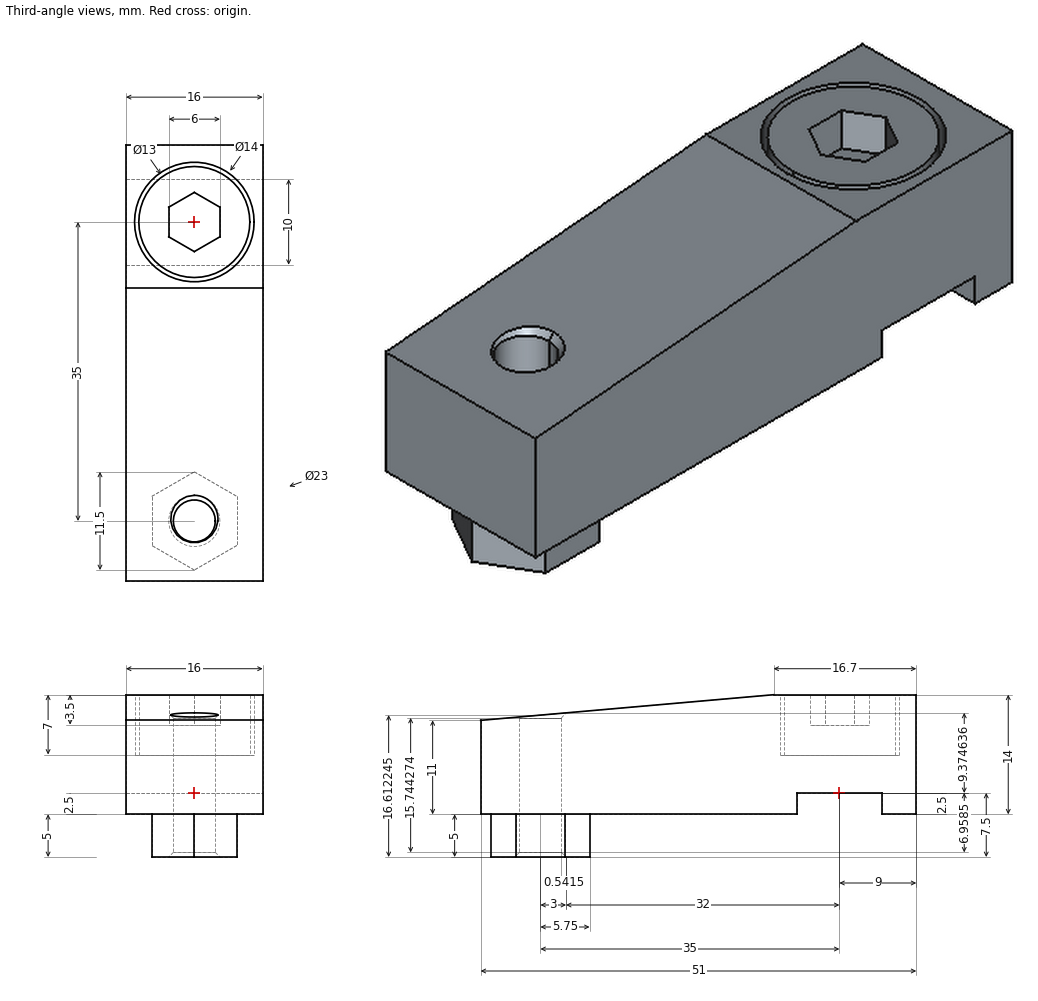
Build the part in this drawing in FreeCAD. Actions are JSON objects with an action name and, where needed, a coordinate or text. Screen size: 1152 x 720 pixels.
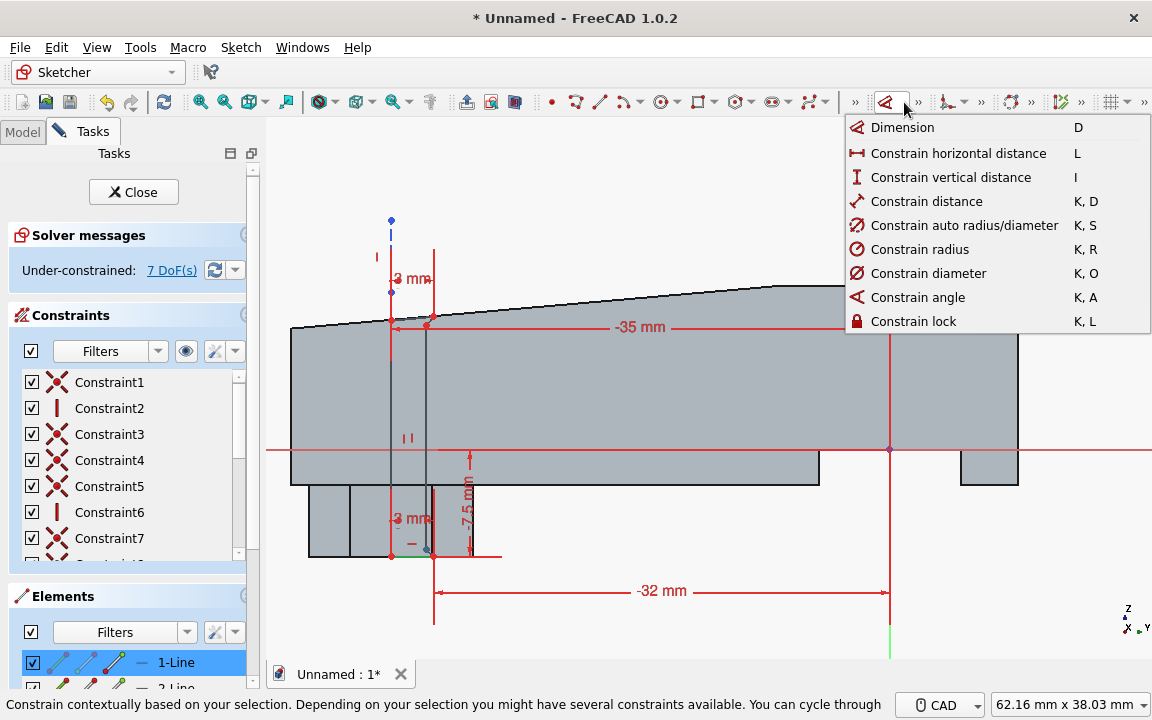
{"action": "left_click", "coordinate": [998, 177]}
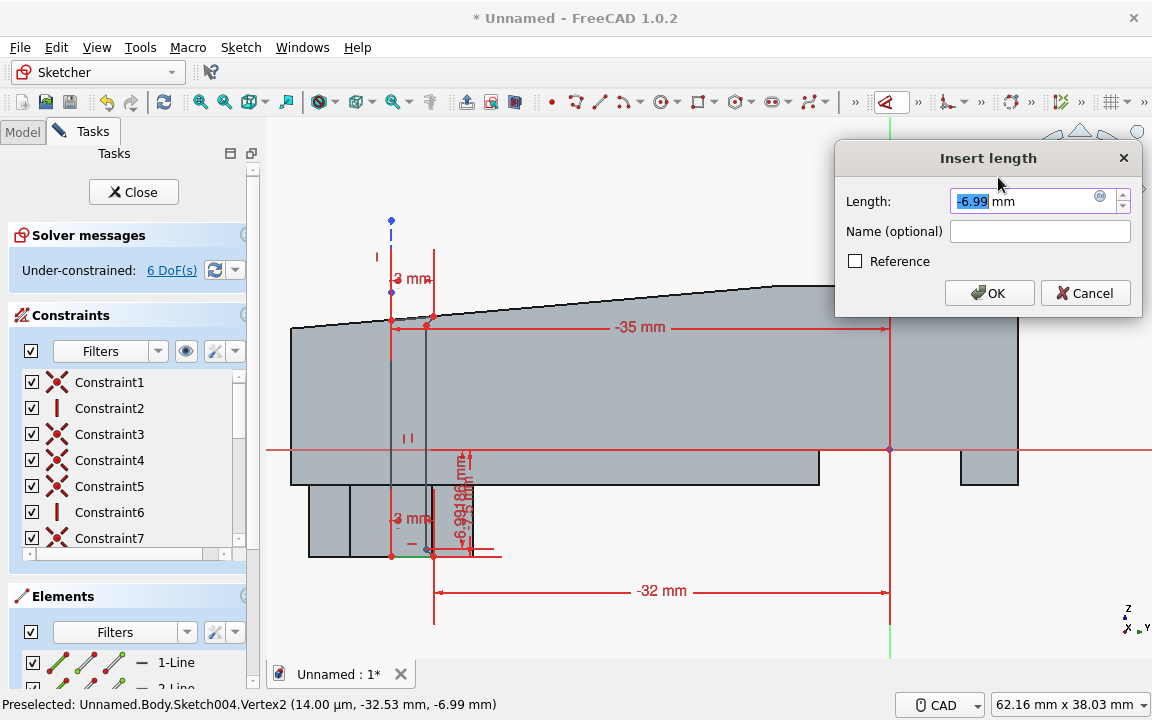
{"action": "type", "text": "-6.9585"}
{"action": "key", "text": "Return"}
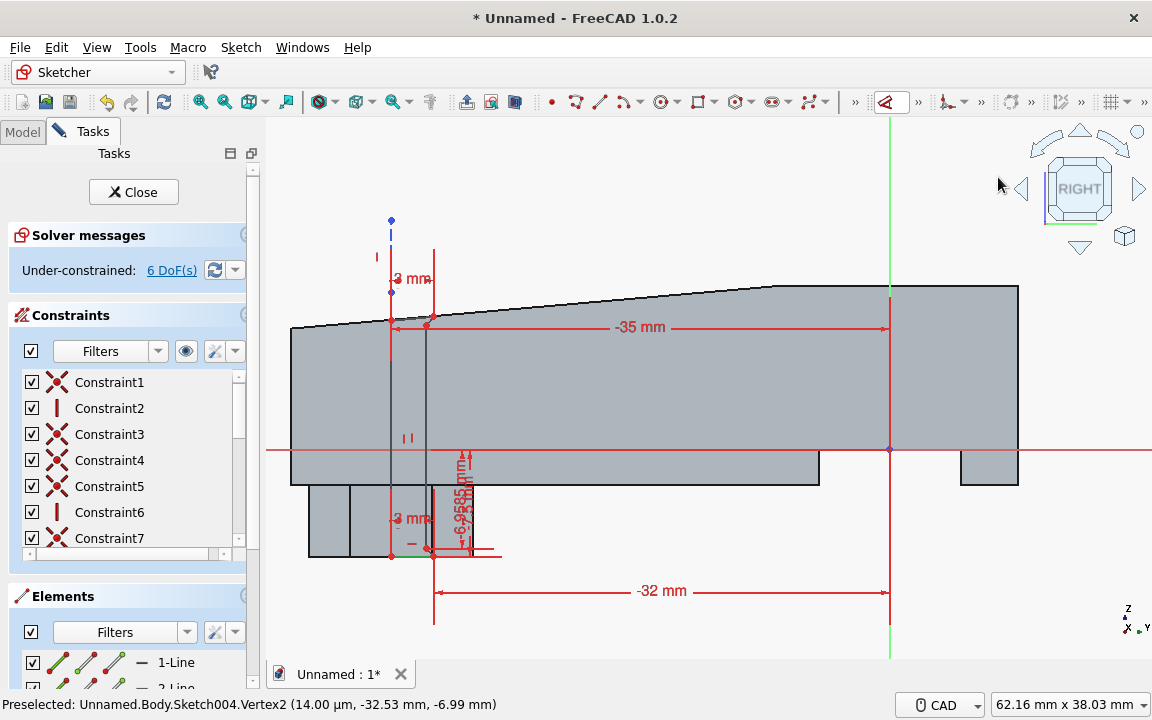
{"action": "scroll", "coordinate": [429, 552], "scroll_direction": "up", "scroll_amount": 9}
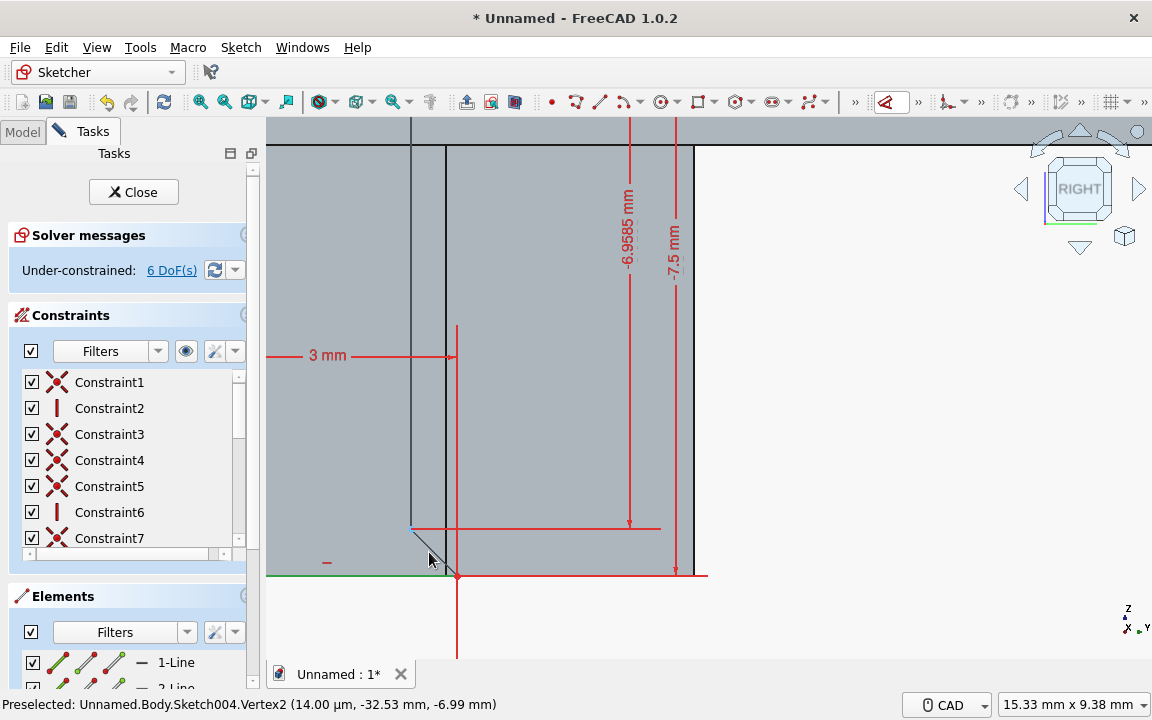
{"action": "left_click", "coordinate": [429, 548]}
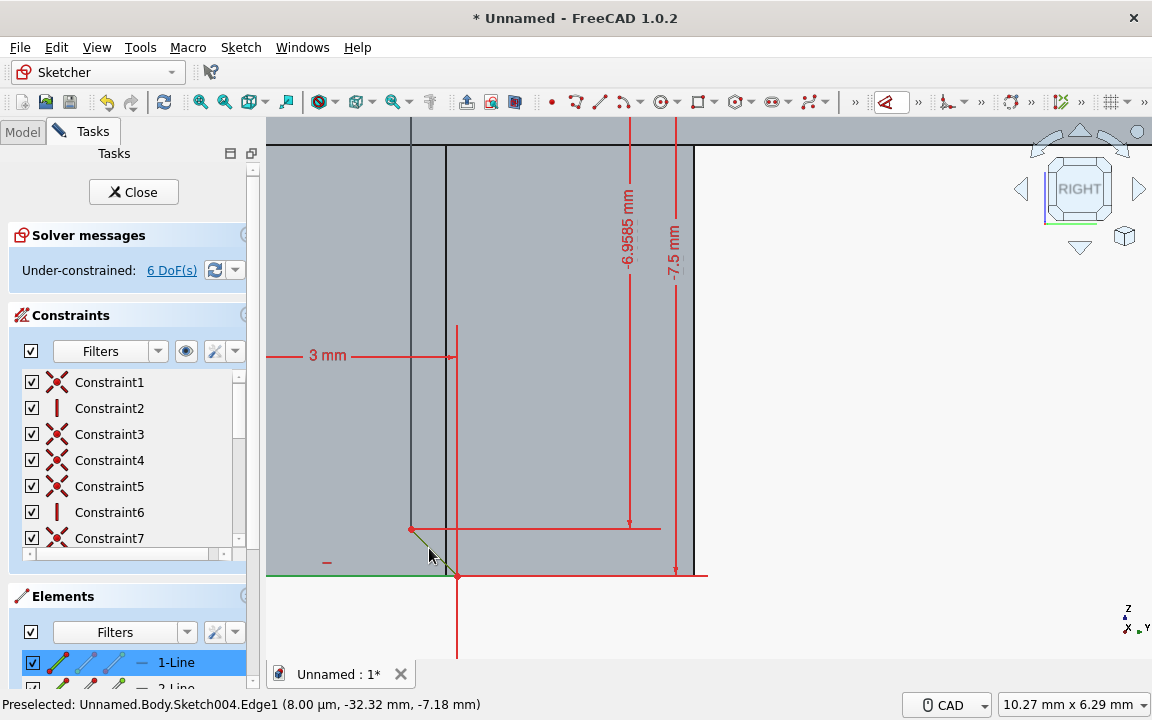
{"action": "key", "text": "l"}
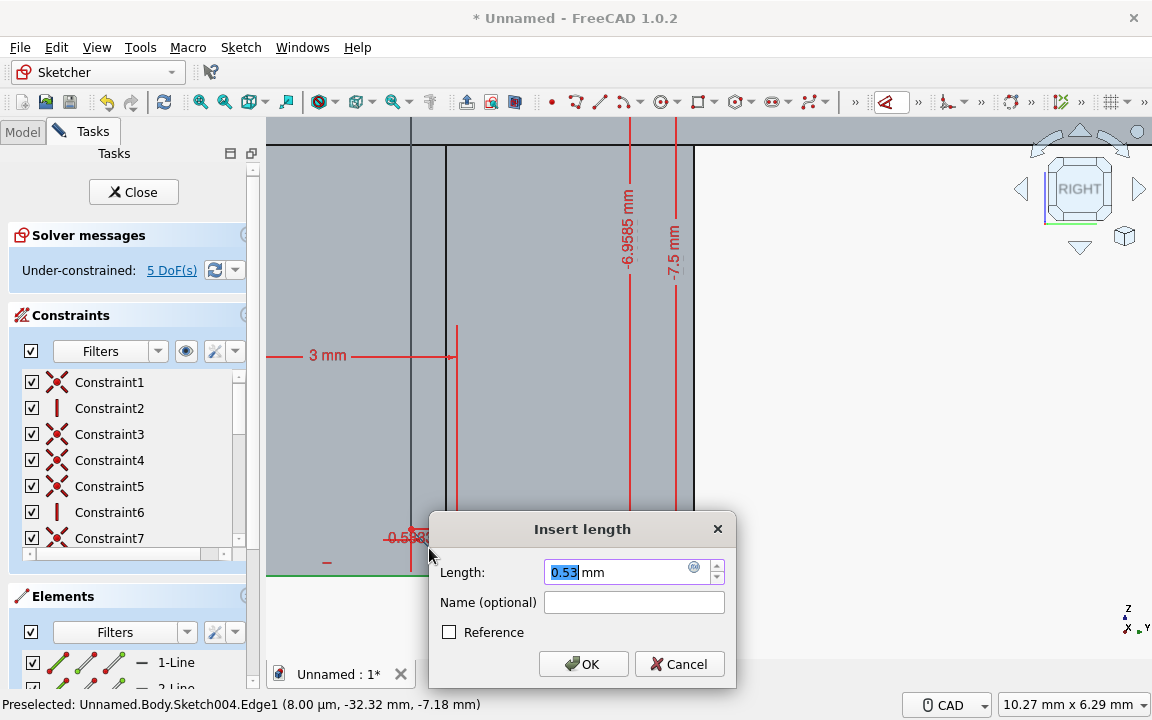
{"action": "type", "text": "0.5415"}
{"action": "key", "text": "Return"}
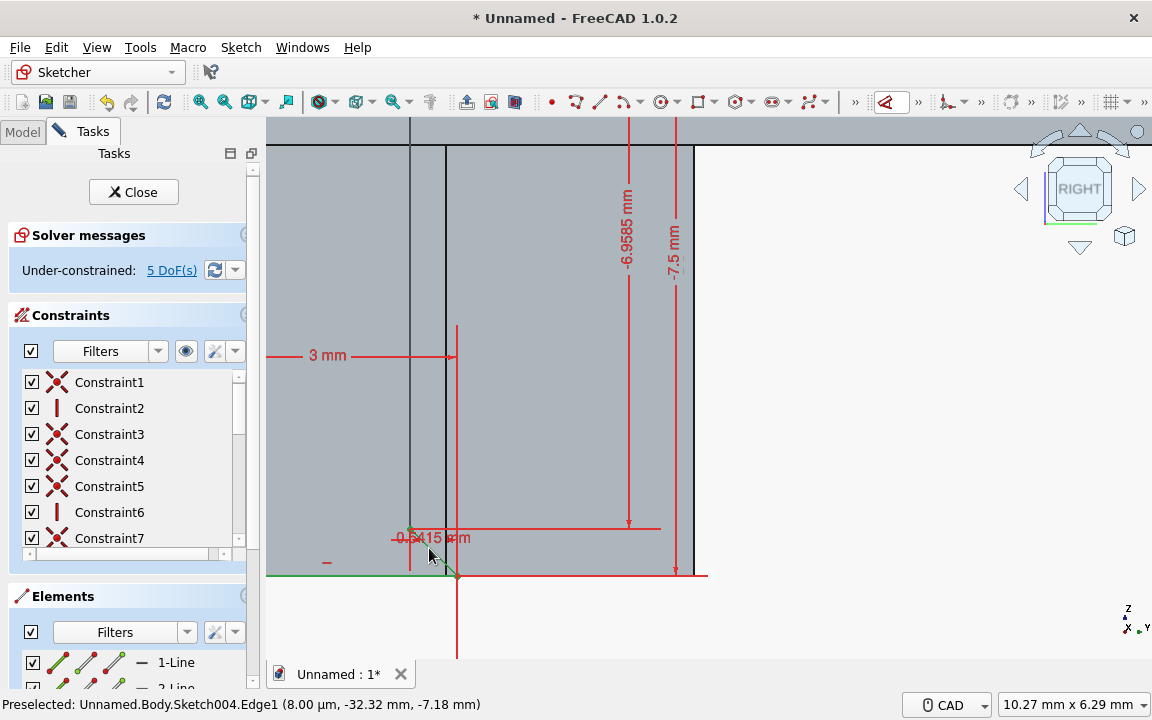
{"action": "scroll", "coordinate": [429, 552], "scroll_direction": "down", "scroll_amount": 9}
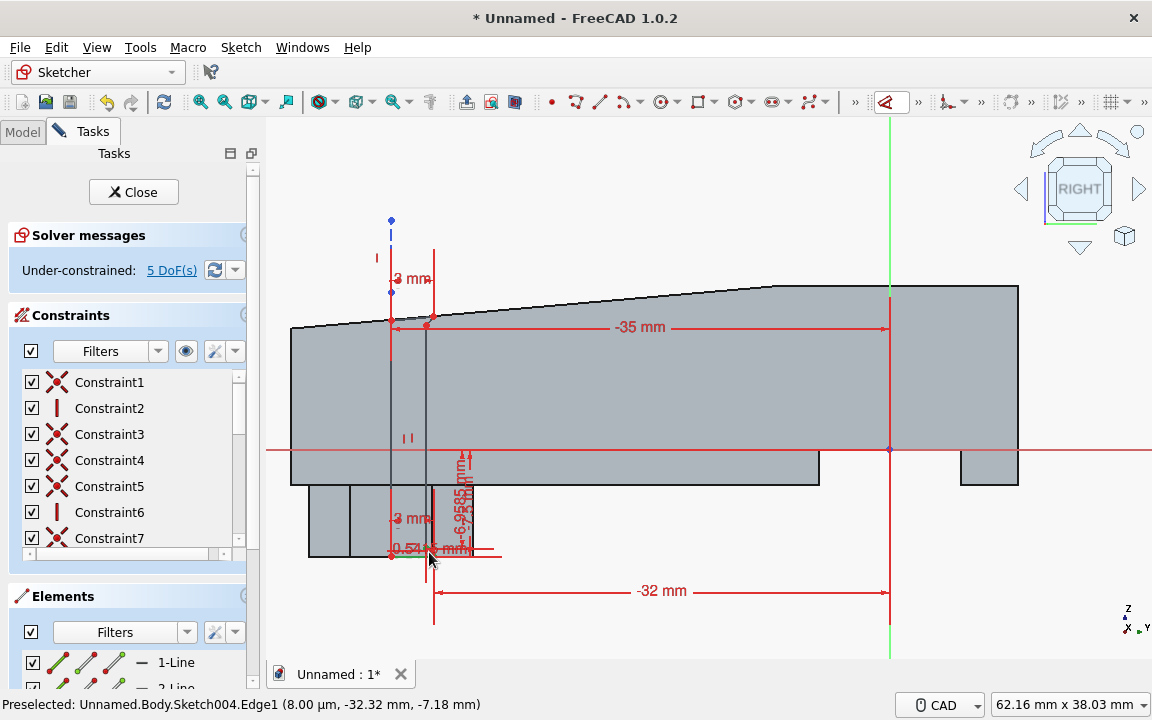
{"action": "left_click", "coordinate": [426, 504]}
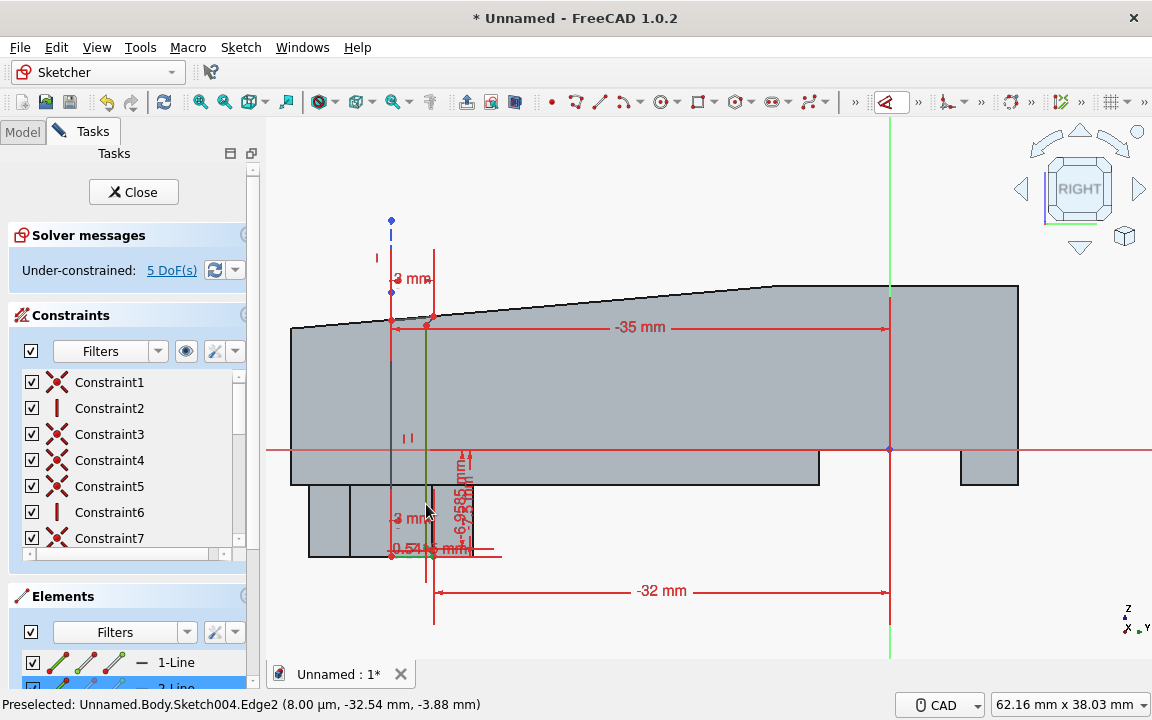
{"action": "key", "text": "i"}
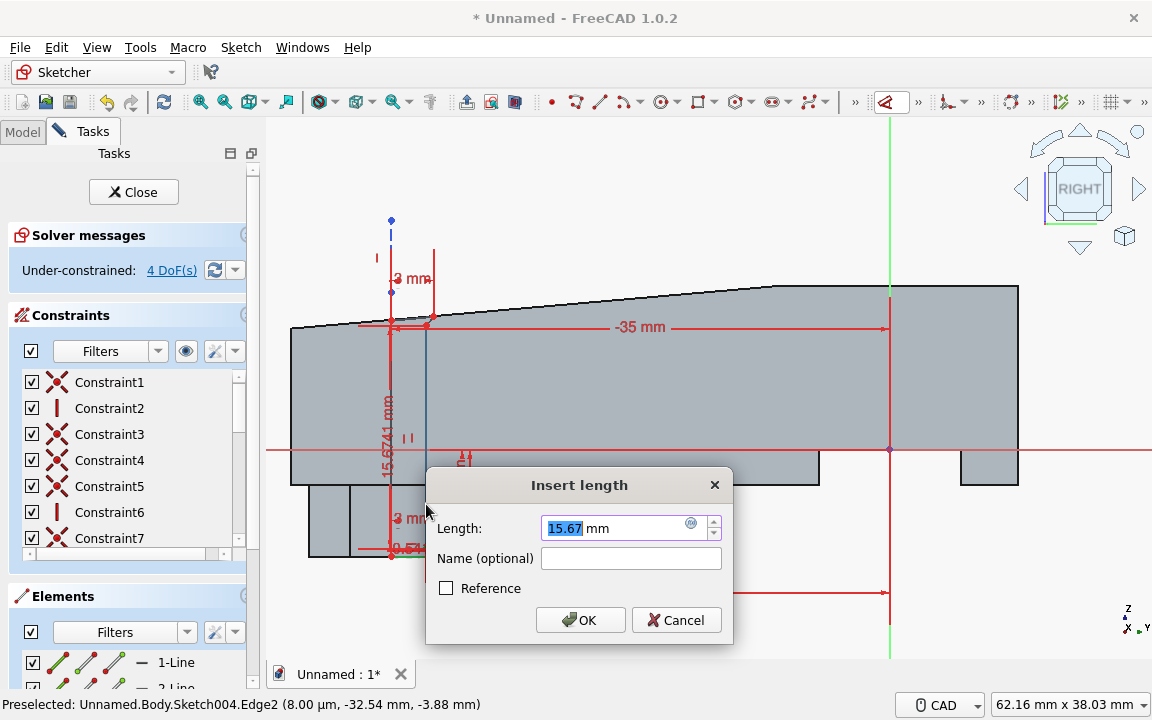
{"action": "type", "text": "15.744274"}
{"action": "key", "text": "Return"}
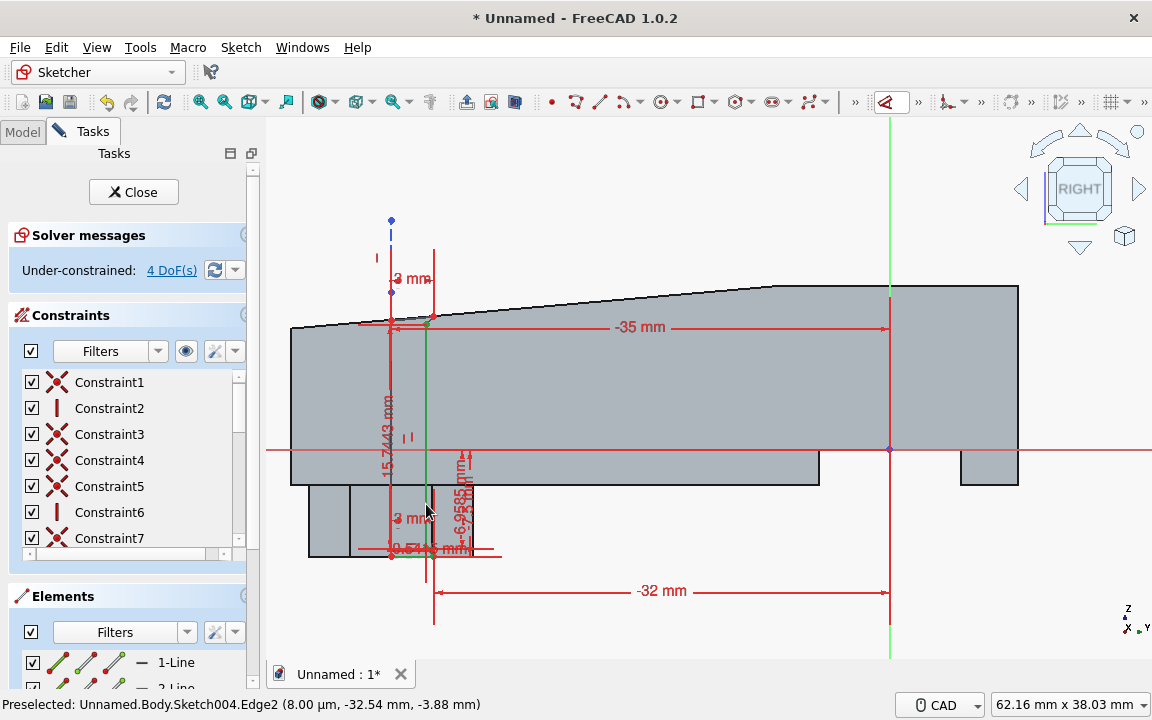
{"action": "left_click", "coordinate": [391, 392]}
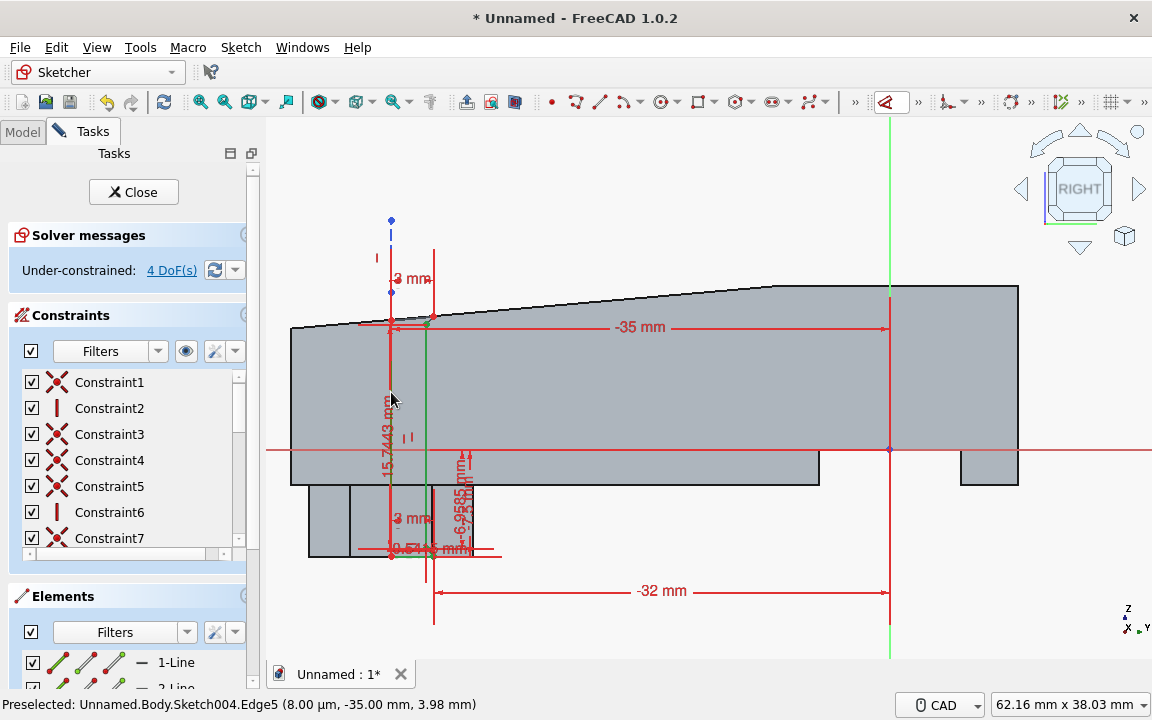
{"action": "left_click", "coordinate": [904, 102]}